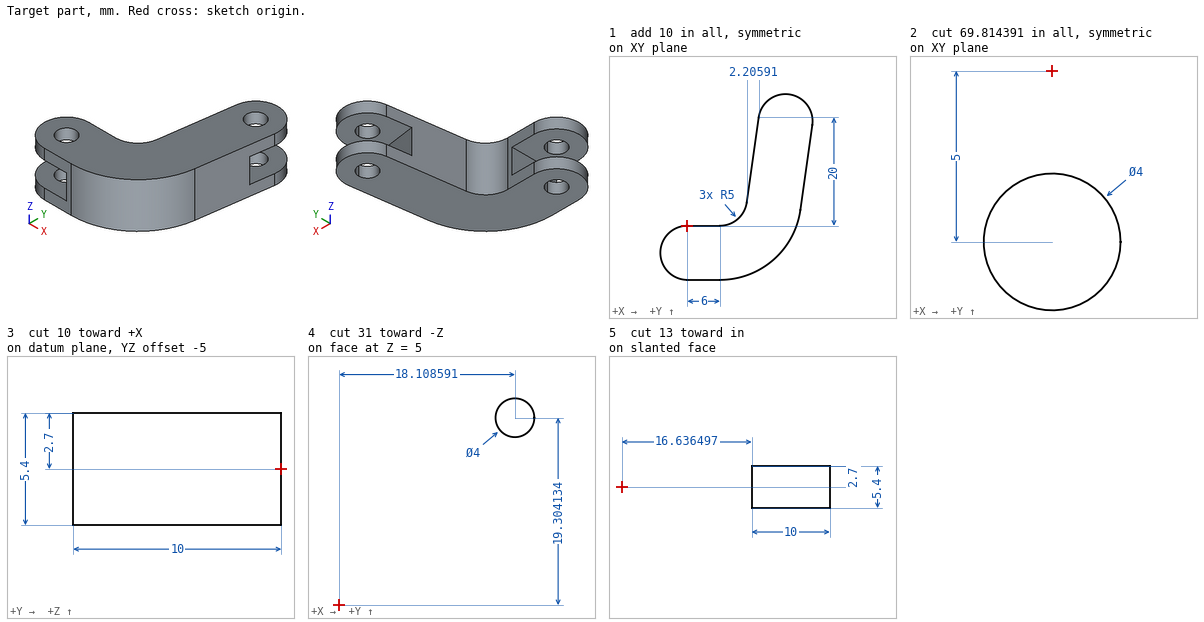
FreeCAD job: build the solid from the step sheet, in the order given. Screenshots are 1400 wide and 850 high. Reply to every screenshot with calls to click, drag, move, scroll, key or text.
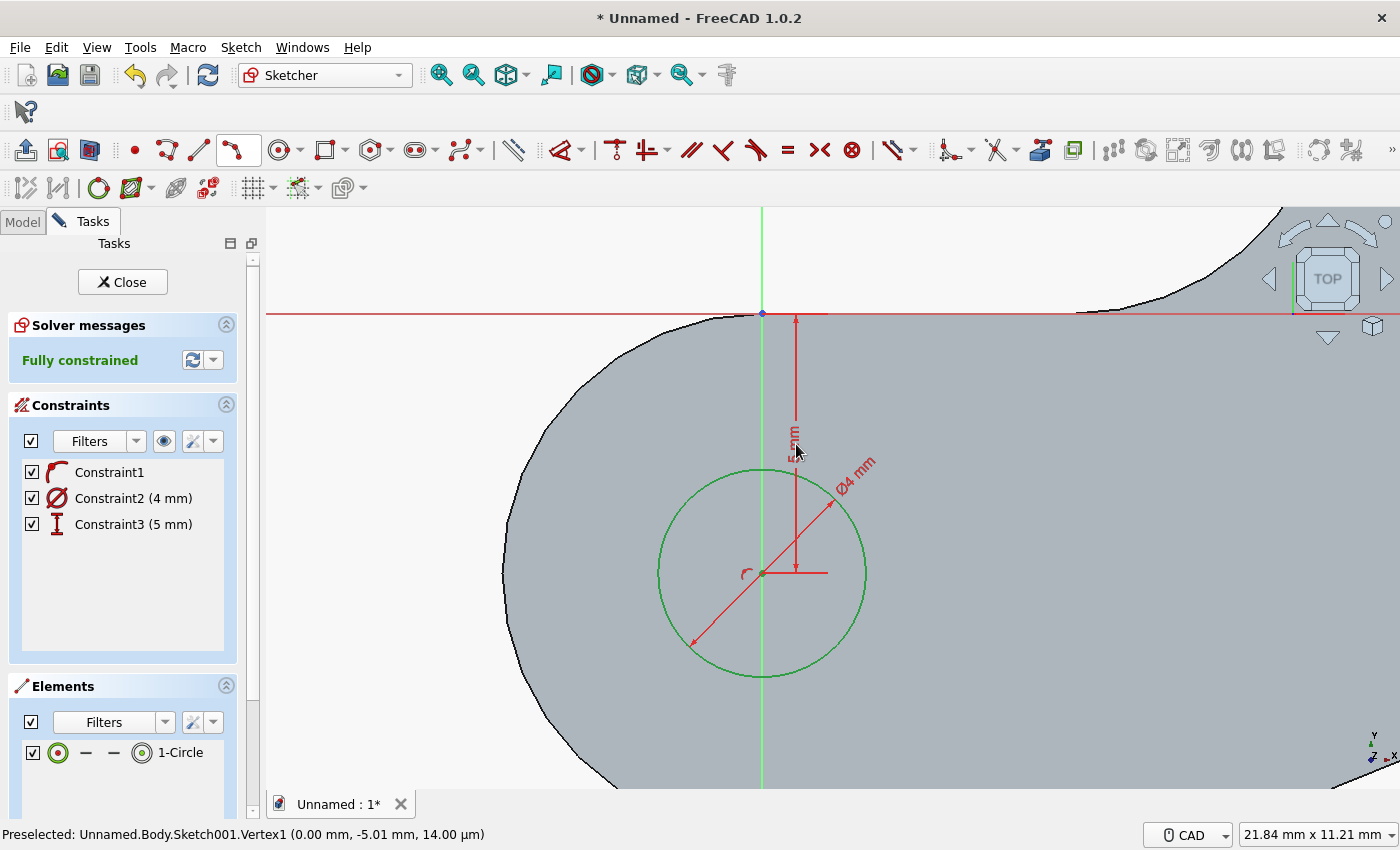
click(123, 282)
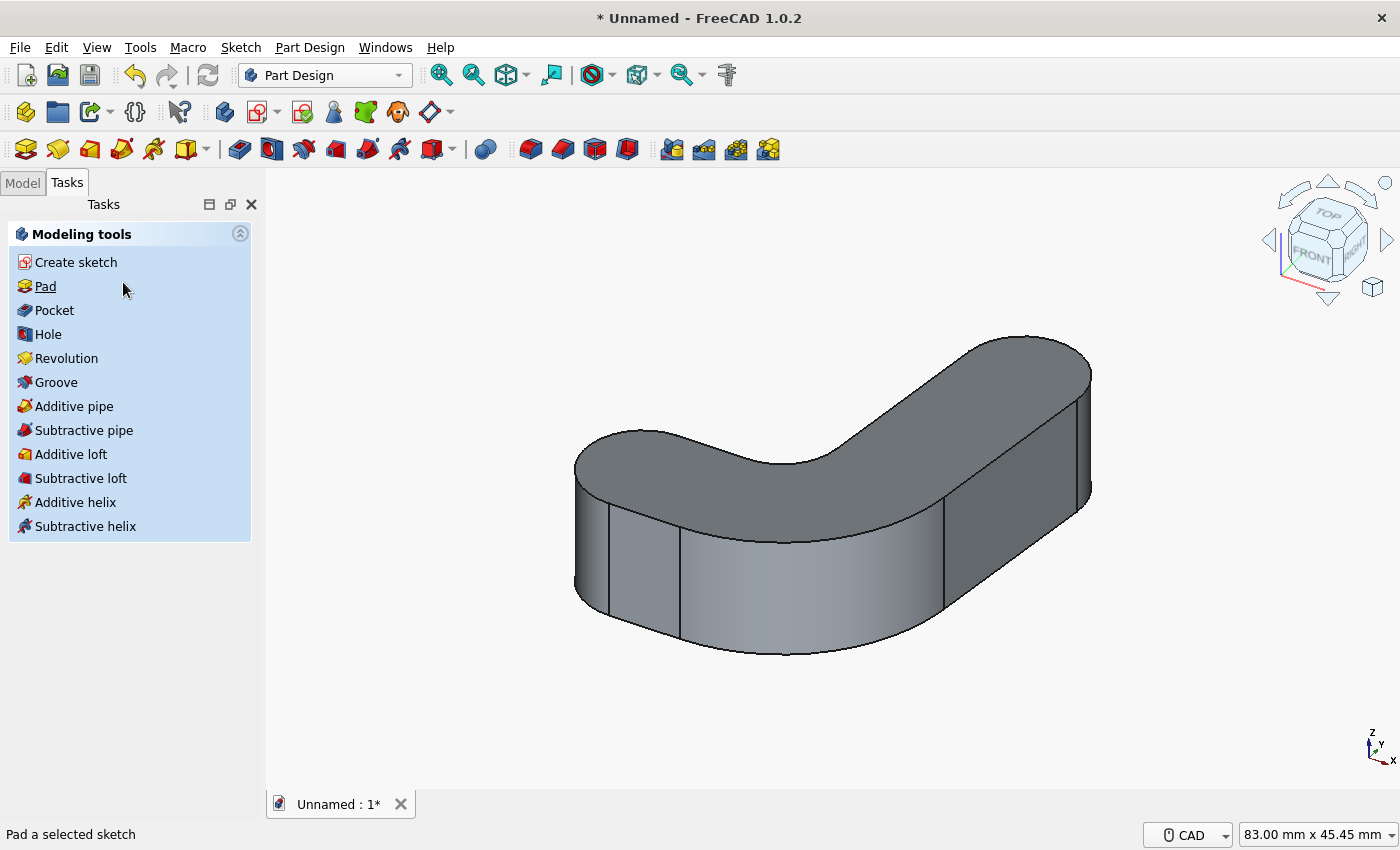
click(240, 150)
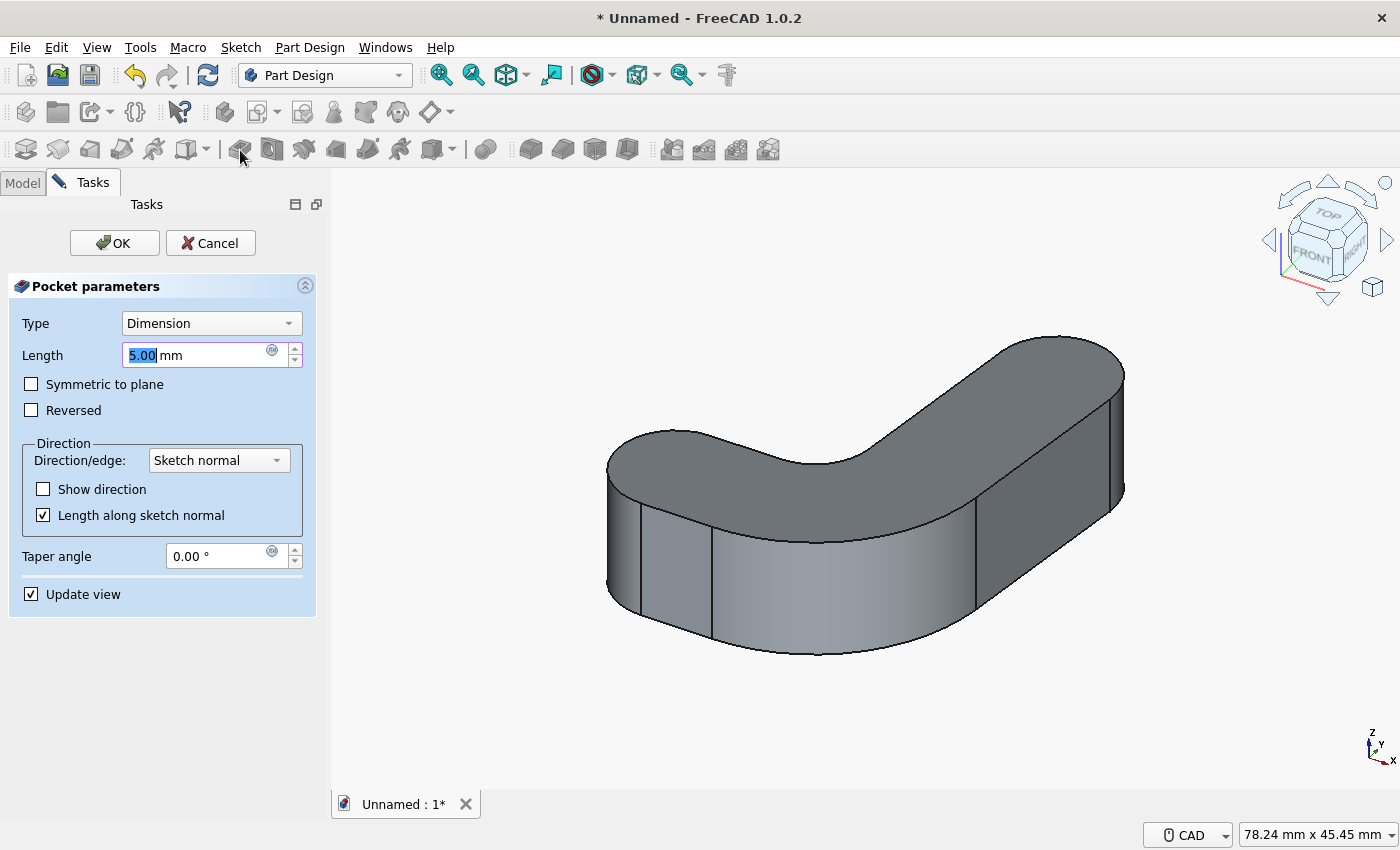
text(69.814391)
key(Tab)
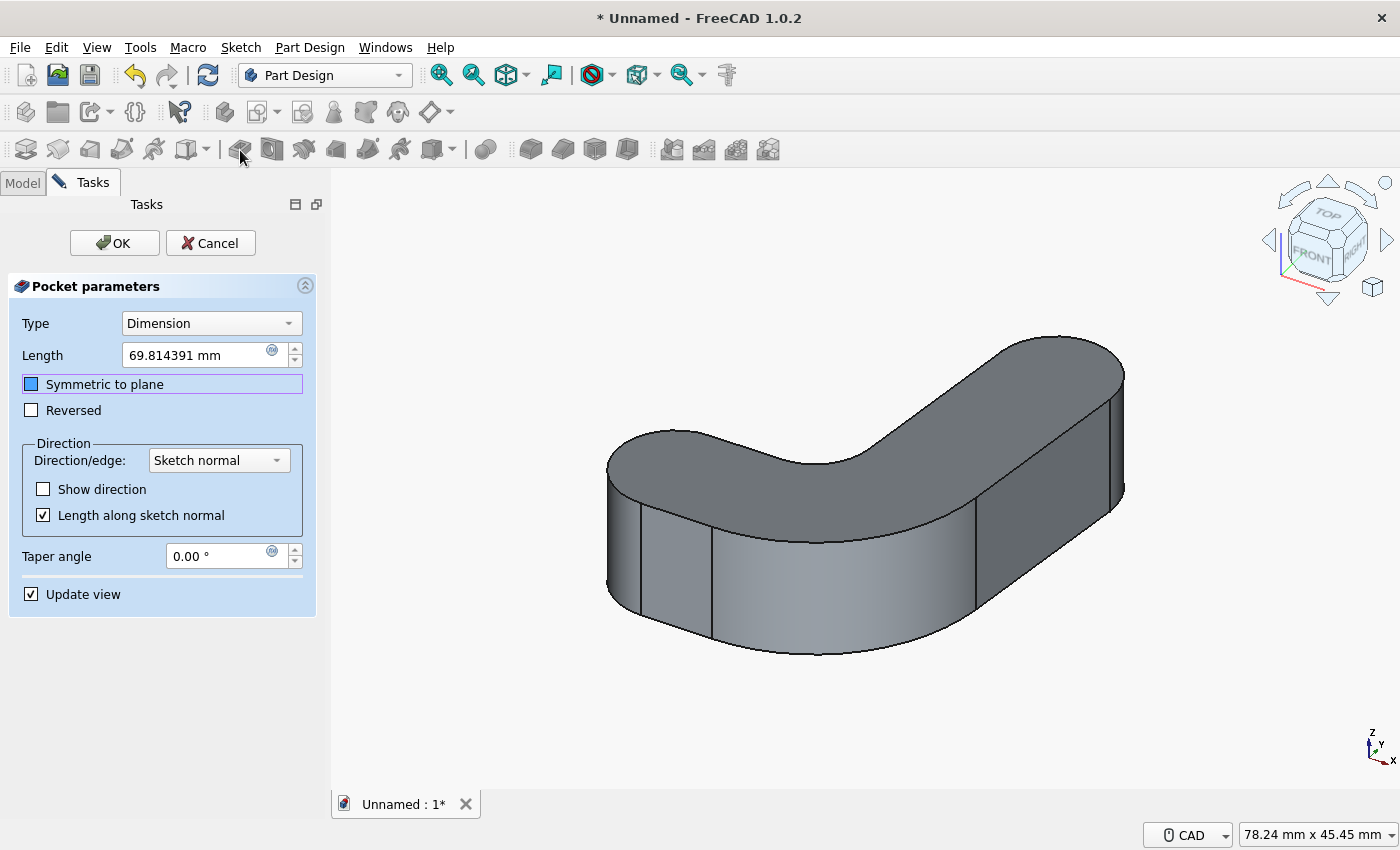
click(30, 384)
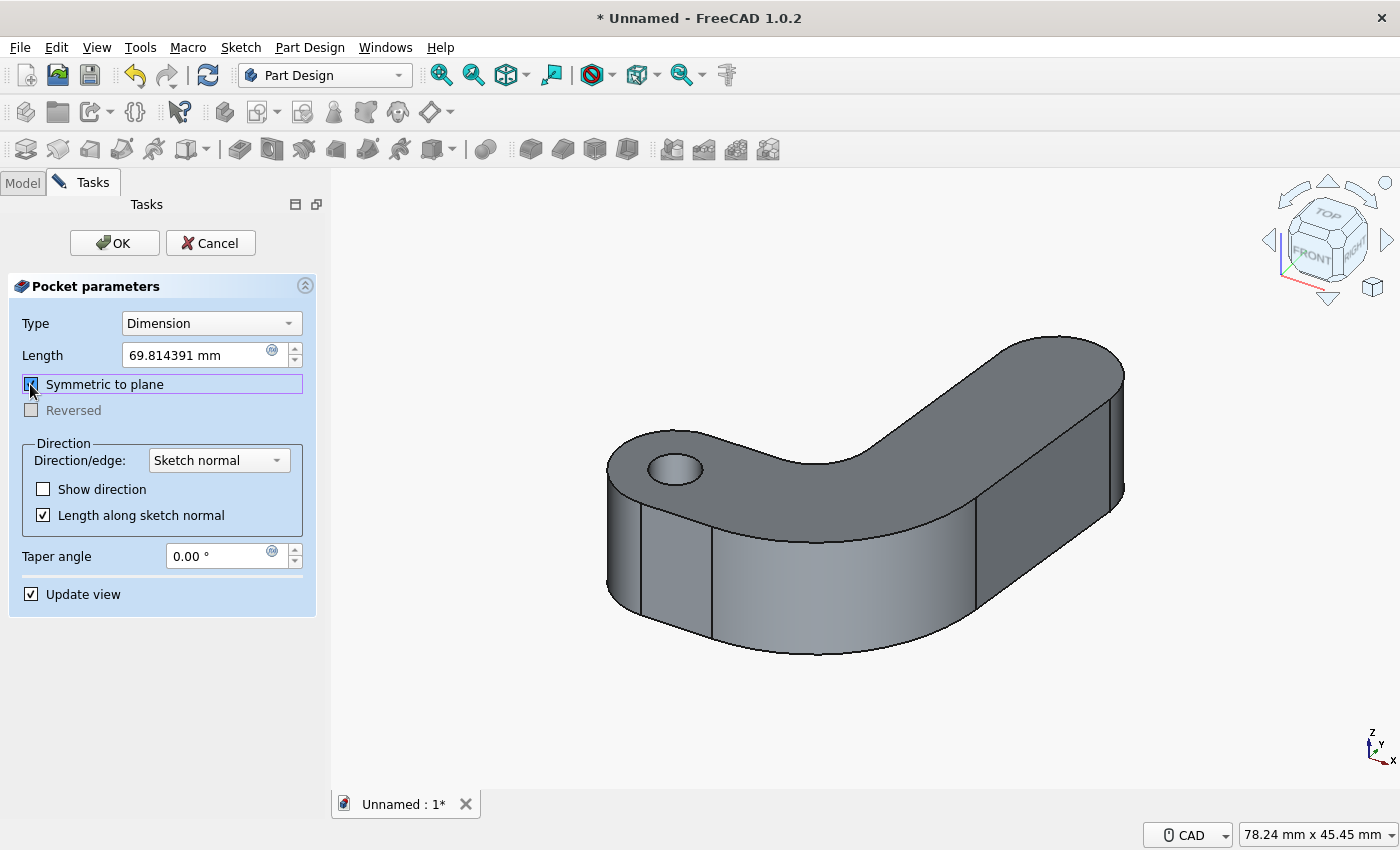
click(115, 243)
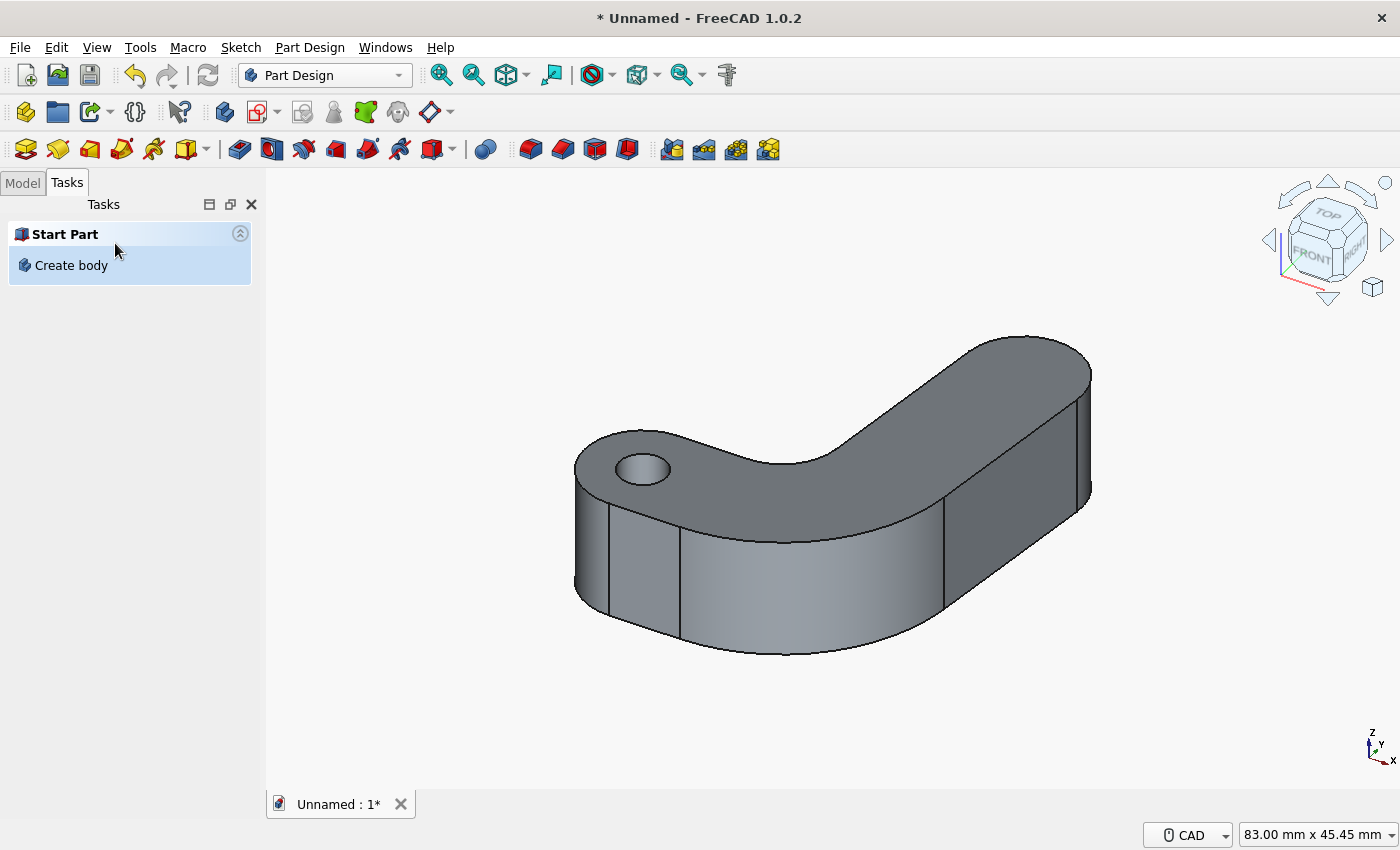
click(23, 182)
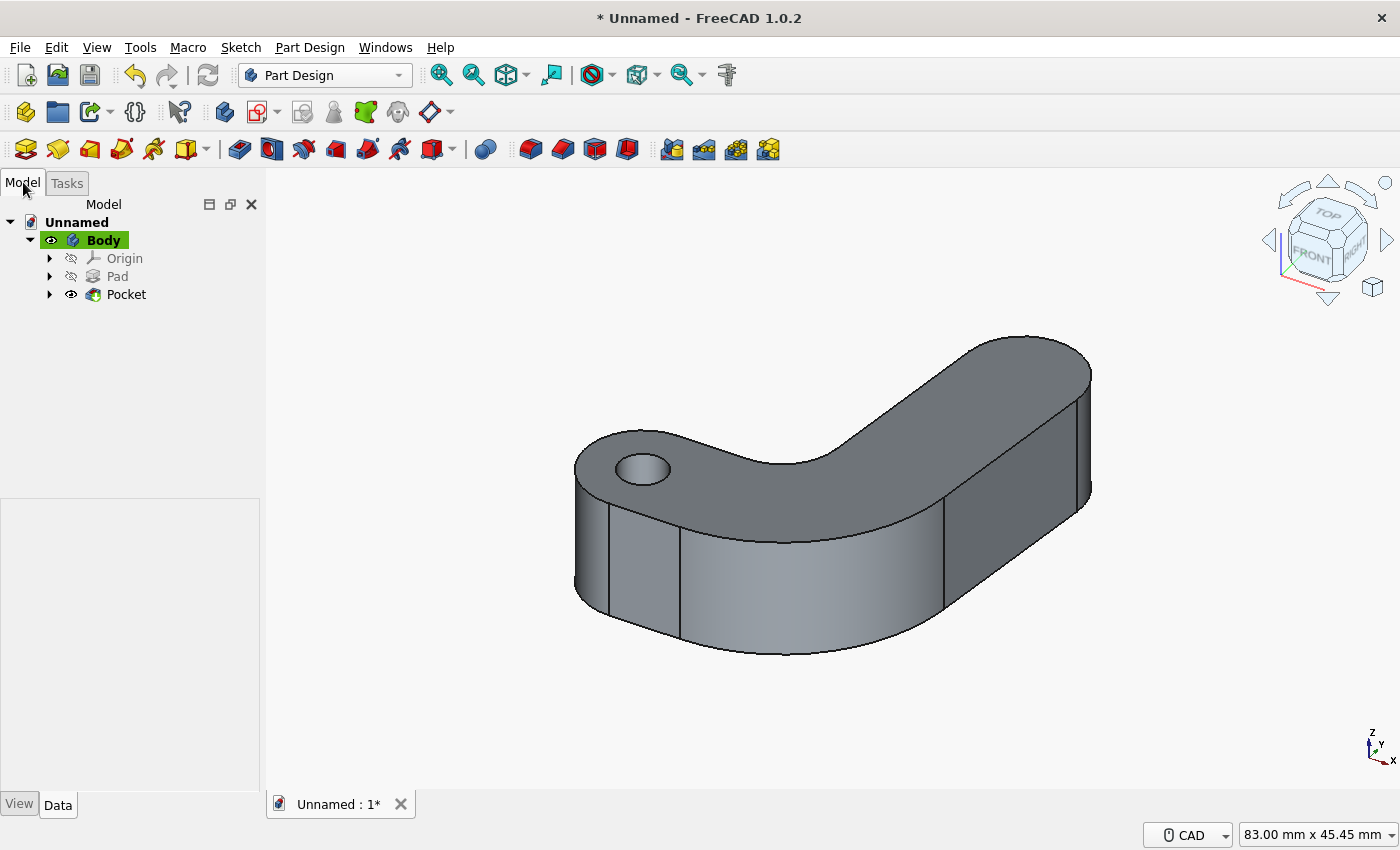
click(50, 258)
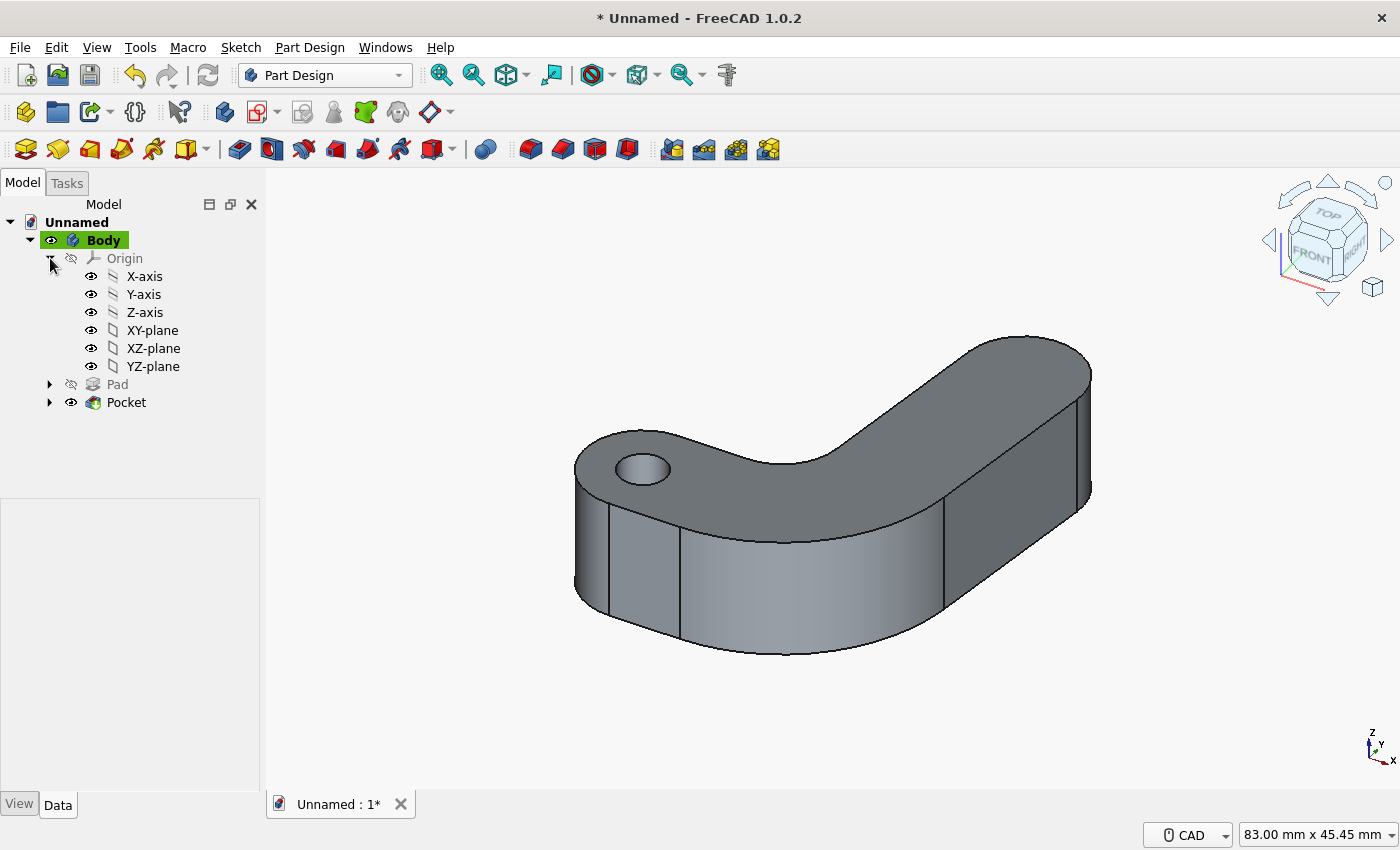
click(136, 366)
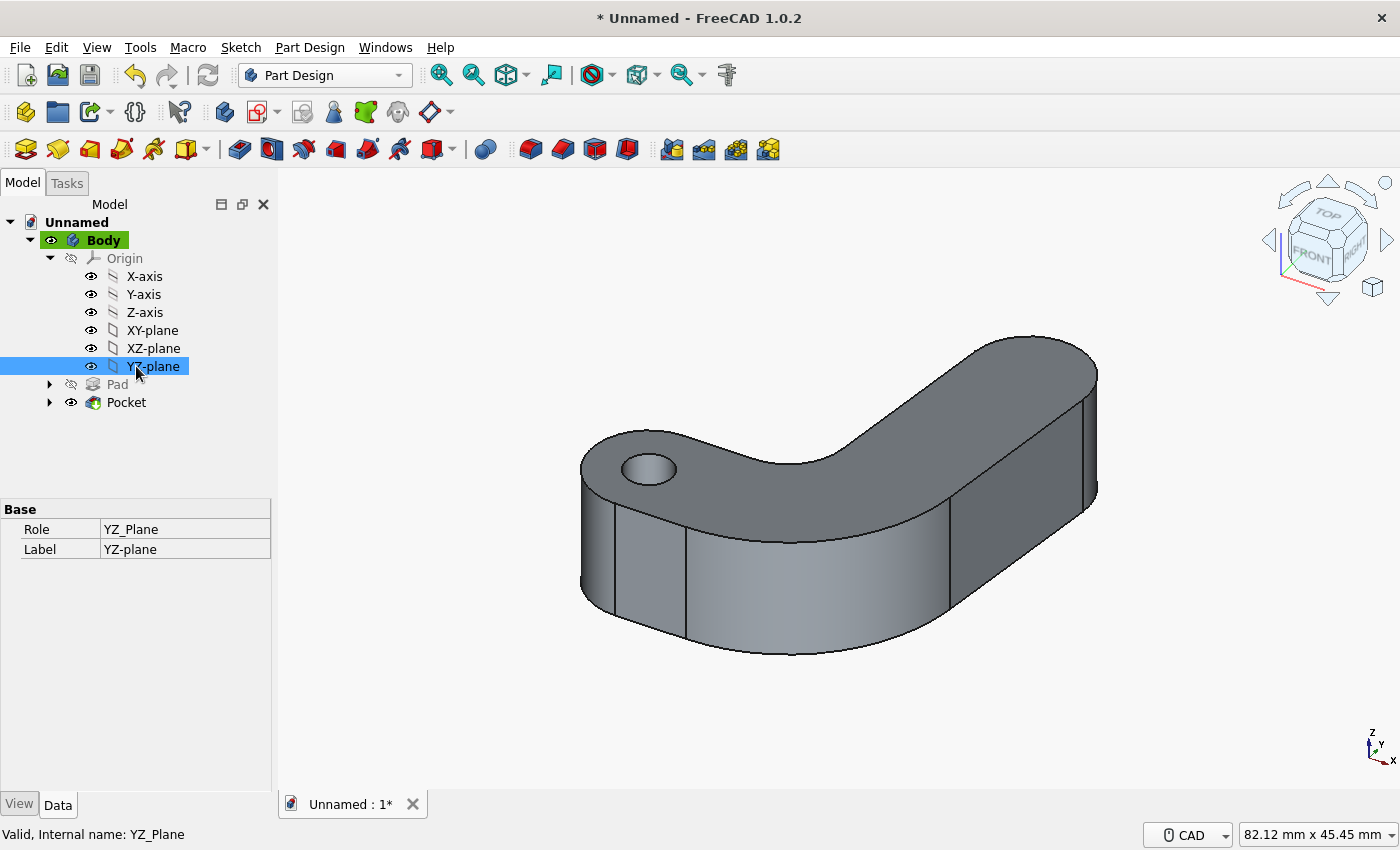
click(430, 112)